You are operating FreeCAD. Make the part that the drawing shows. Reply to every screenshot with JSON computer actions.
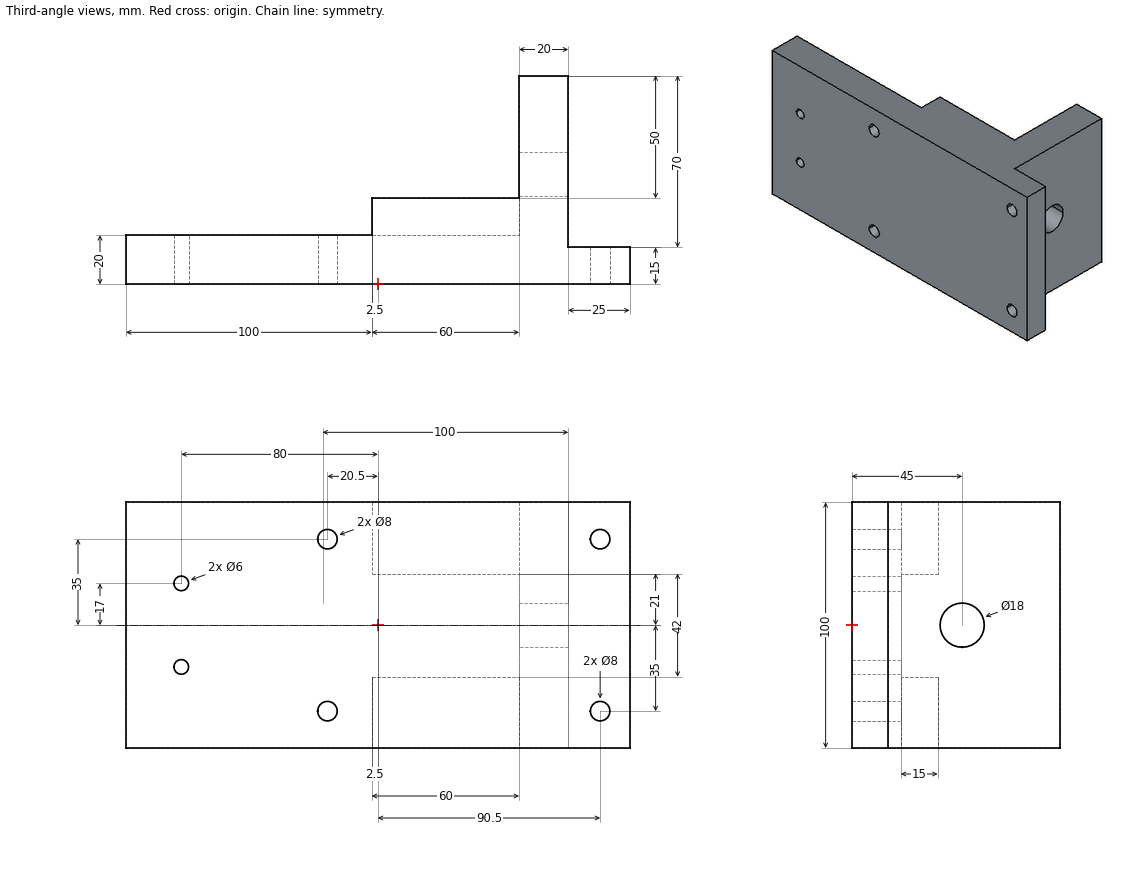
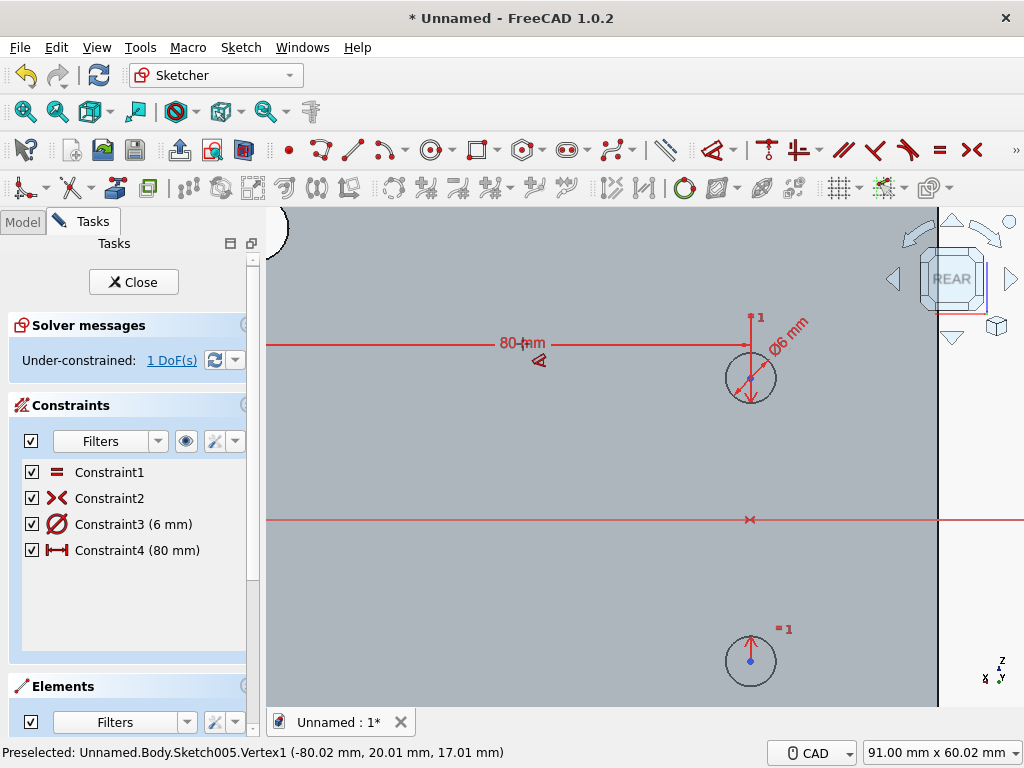
{"action": "left_click", "coordinate": [751, 378]}
{"action": "left_click", "coordinate": [785, 449]}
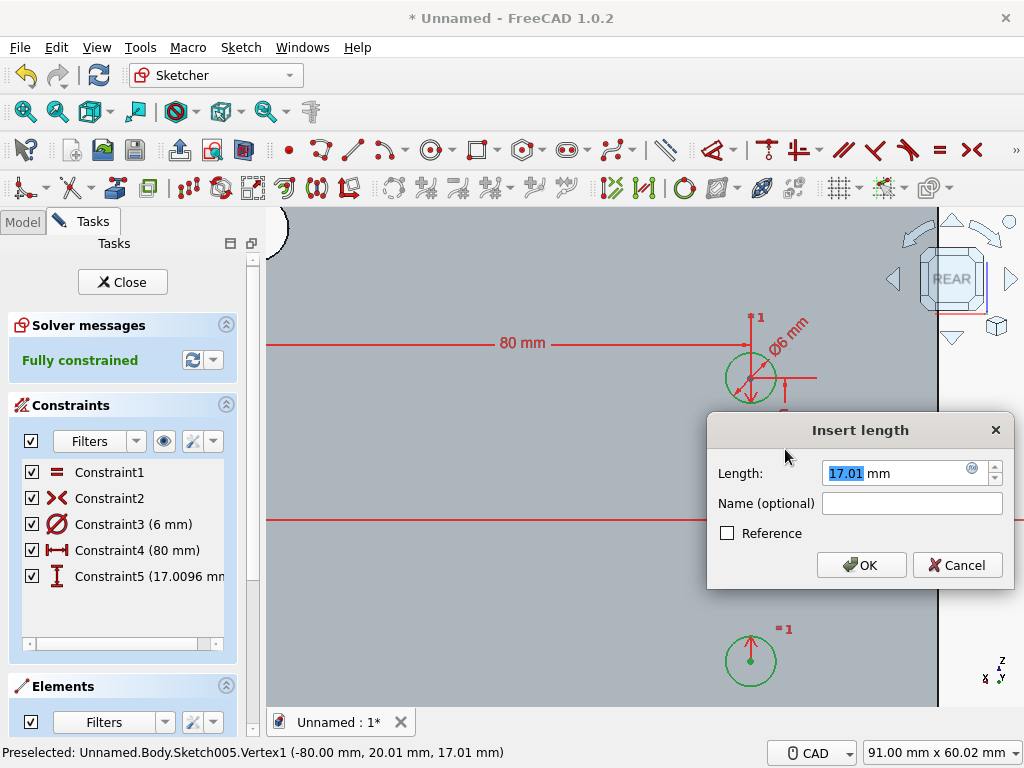
{"action": "type", "text": "17"}
{"action": "key", "text": "Return"}
{"action": "key", "text": "Escape"}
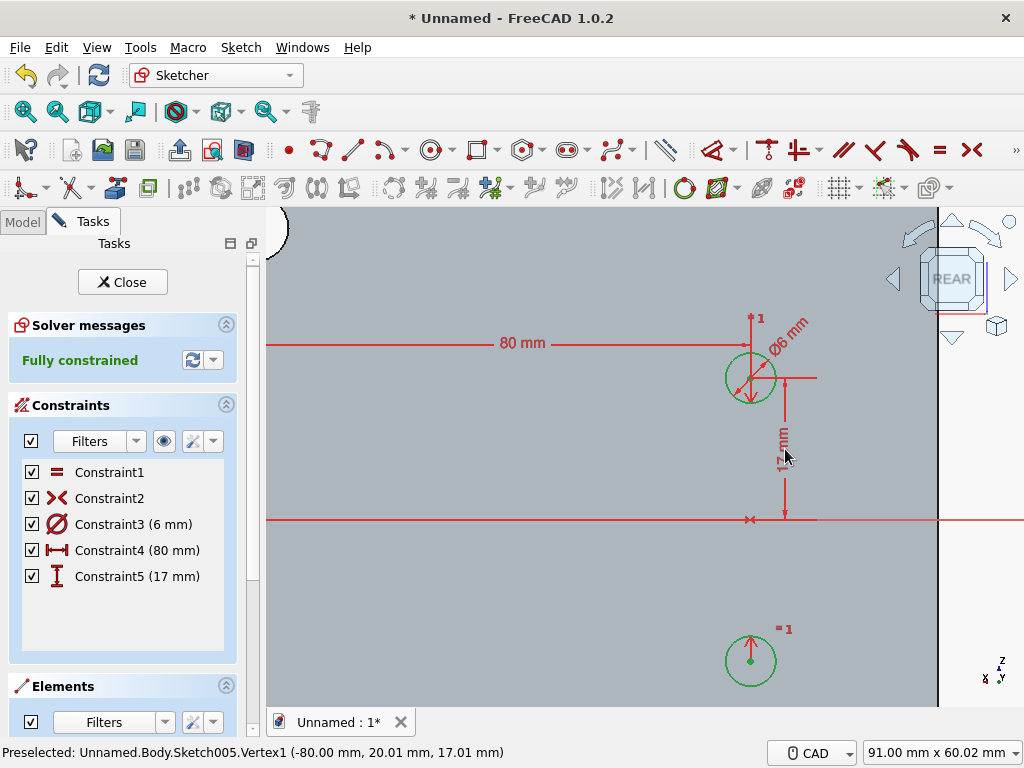
{"action": "left_click", "coordinate": [123, 282]}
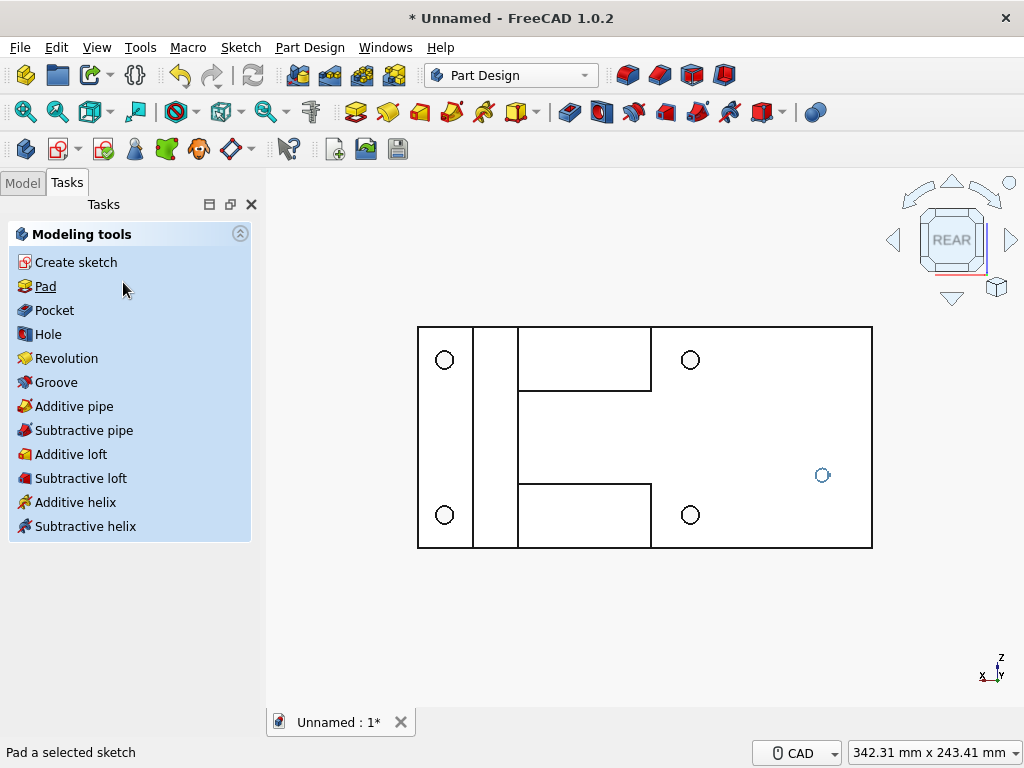
{"action": "left_click", "coordinate": [570, 112]}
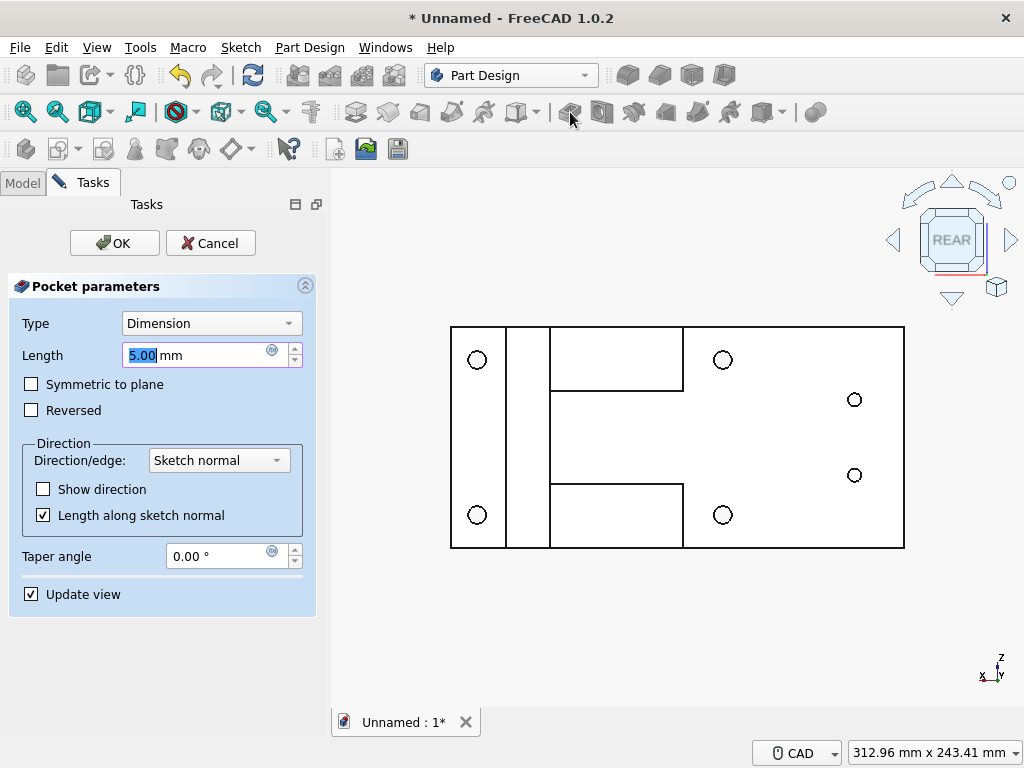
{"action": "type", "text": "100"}
{"action": "key", "text": "Tab"}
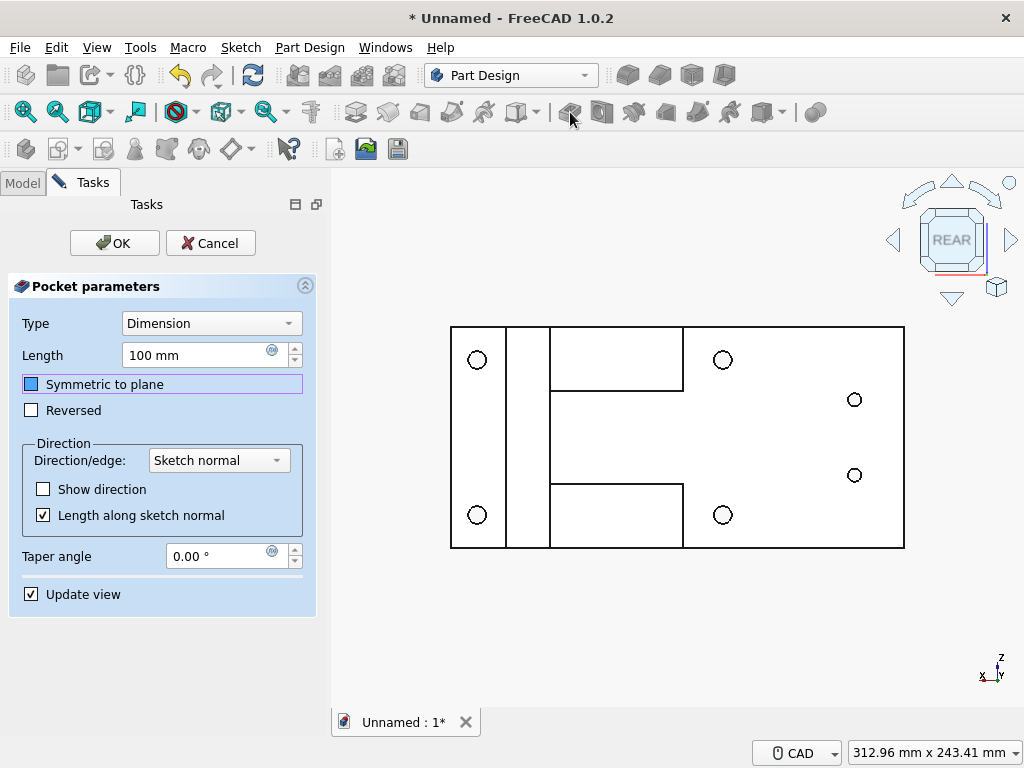
{"action": "left_click", "coordinate": [115, 243]}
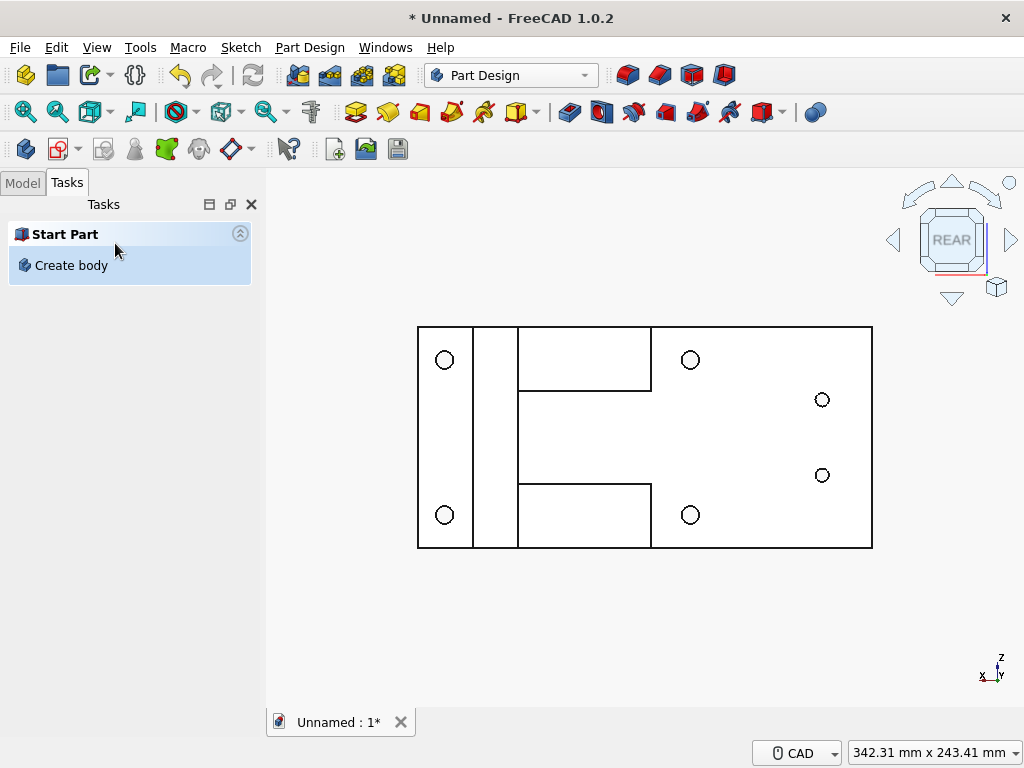
{"action": "key", "text": "0"}